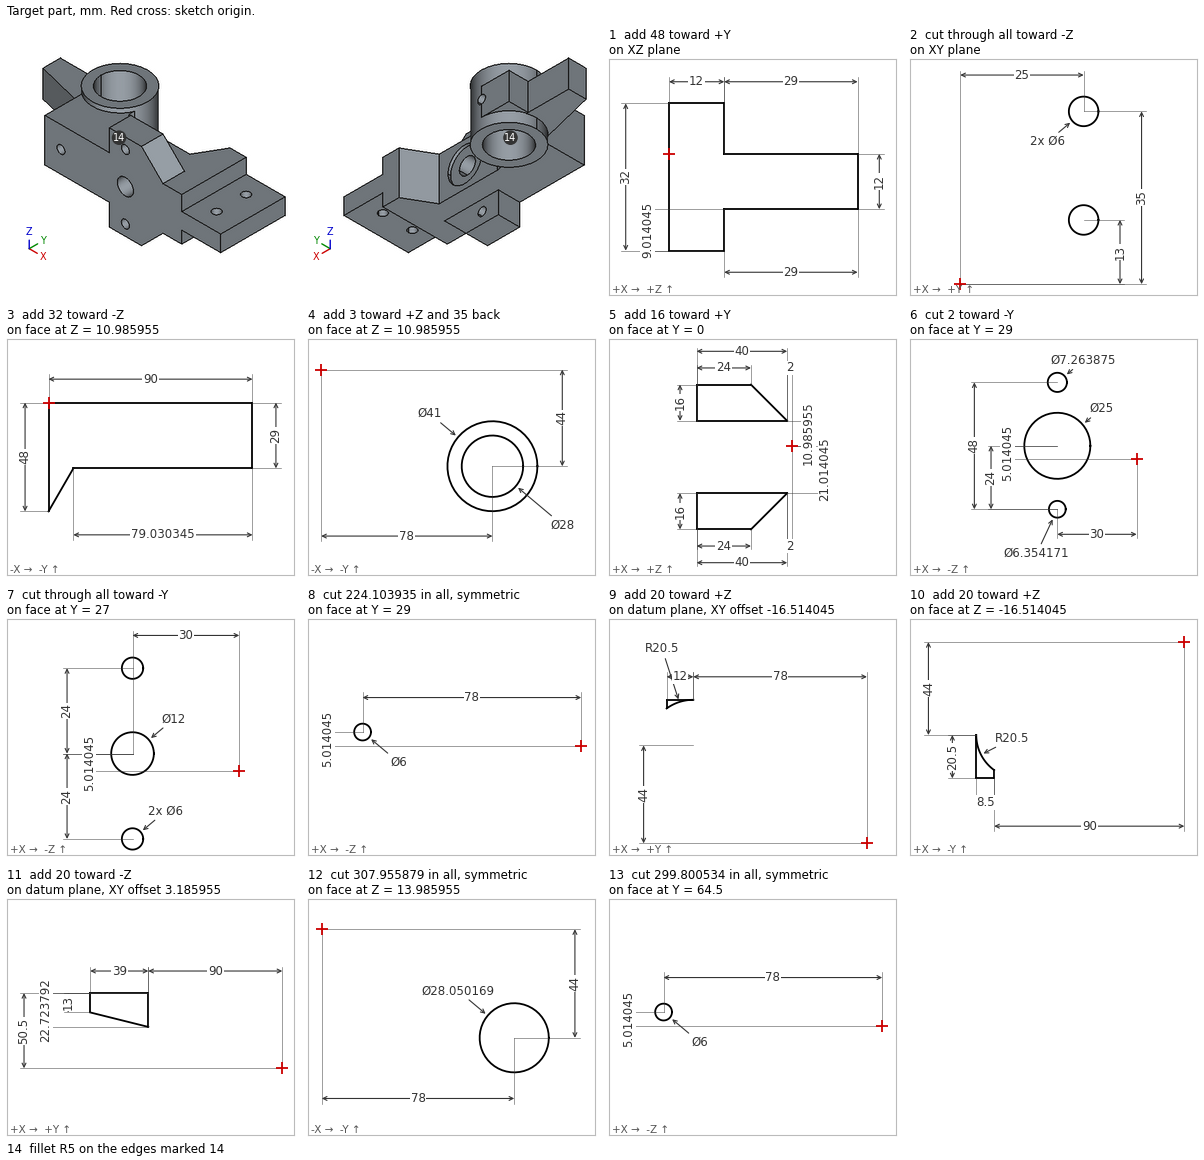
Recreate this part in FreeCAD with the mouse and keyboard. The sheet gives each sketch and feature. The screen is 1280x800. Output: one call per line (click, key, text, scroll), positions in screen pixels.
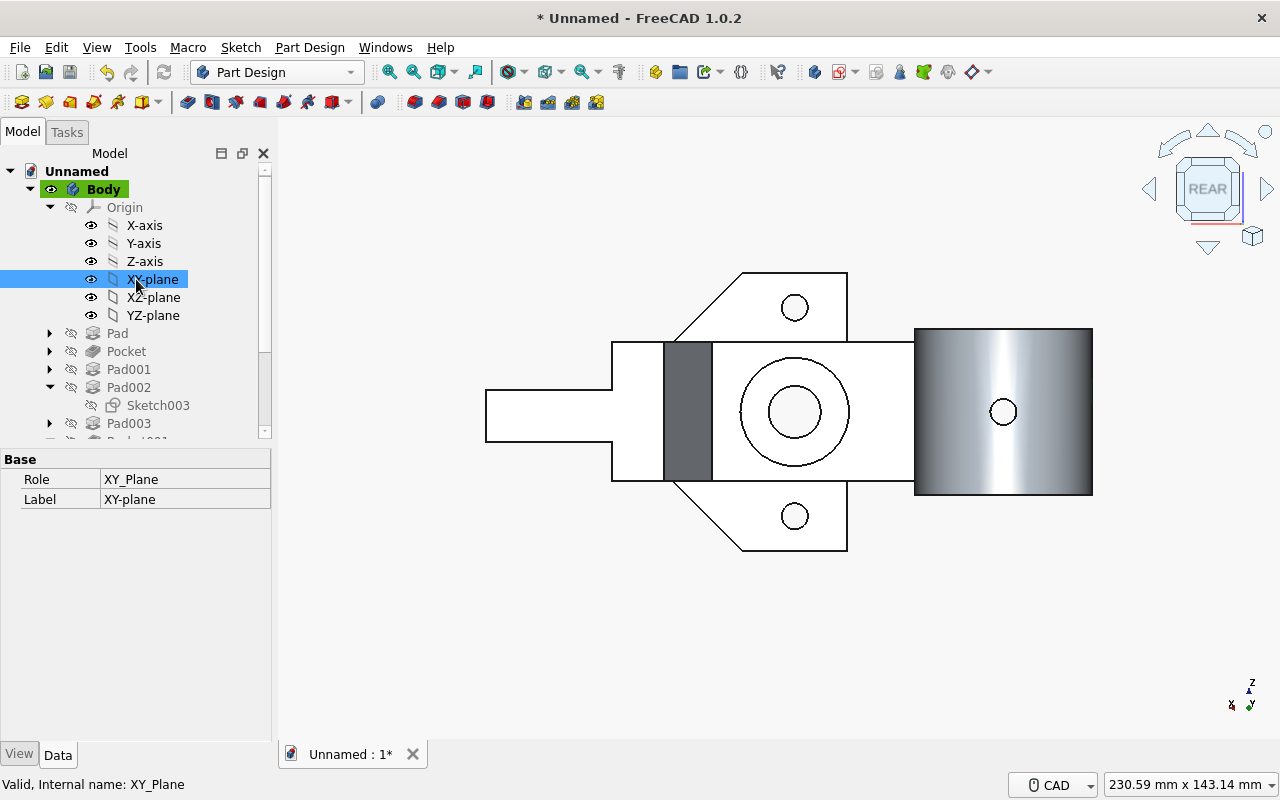
click(972, 72)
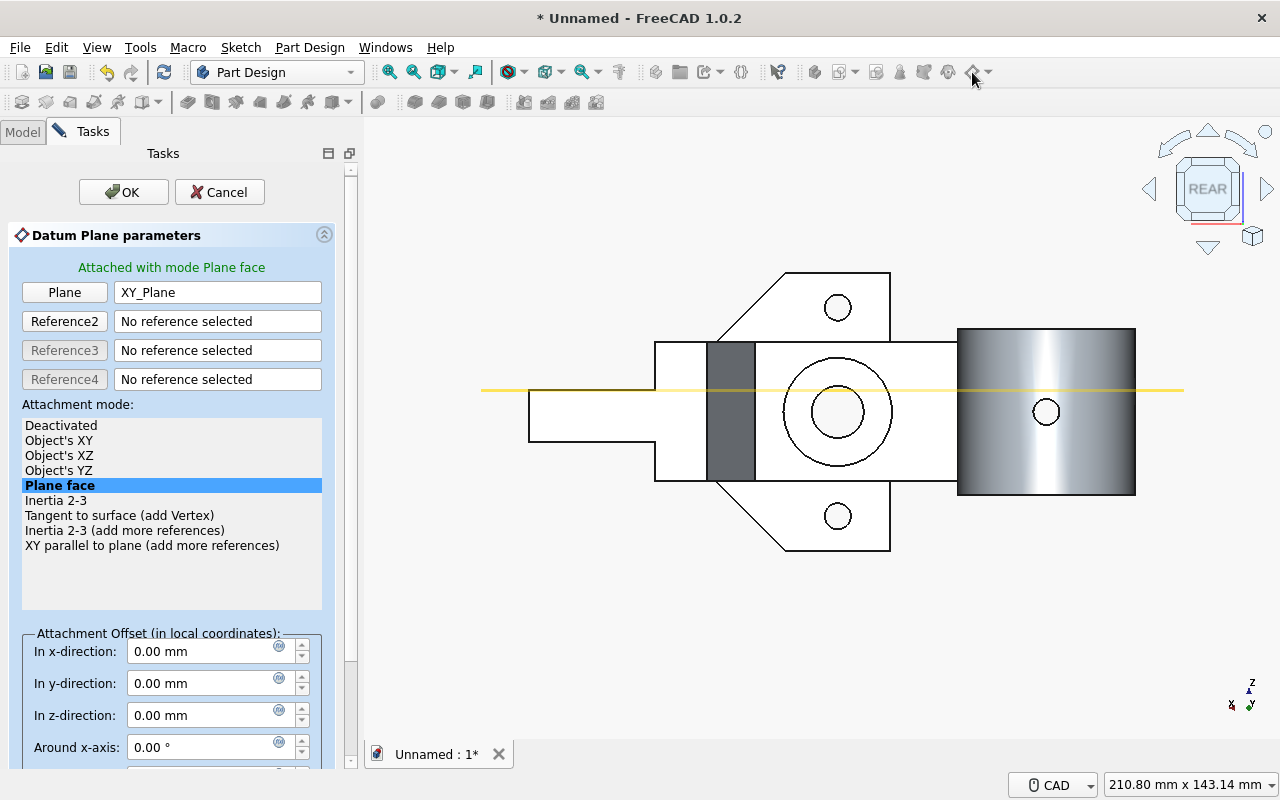
triple_click(210, 715)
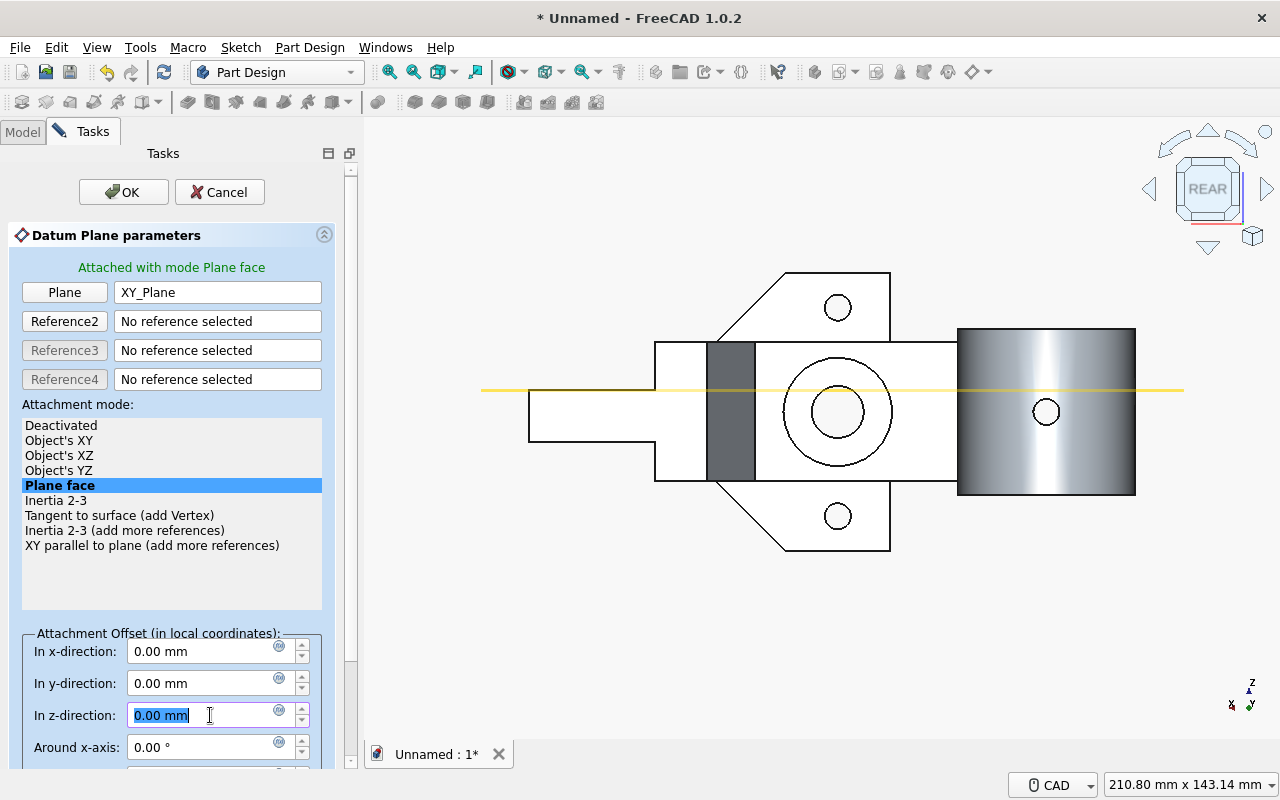
text(-16.514045)
key(Tab)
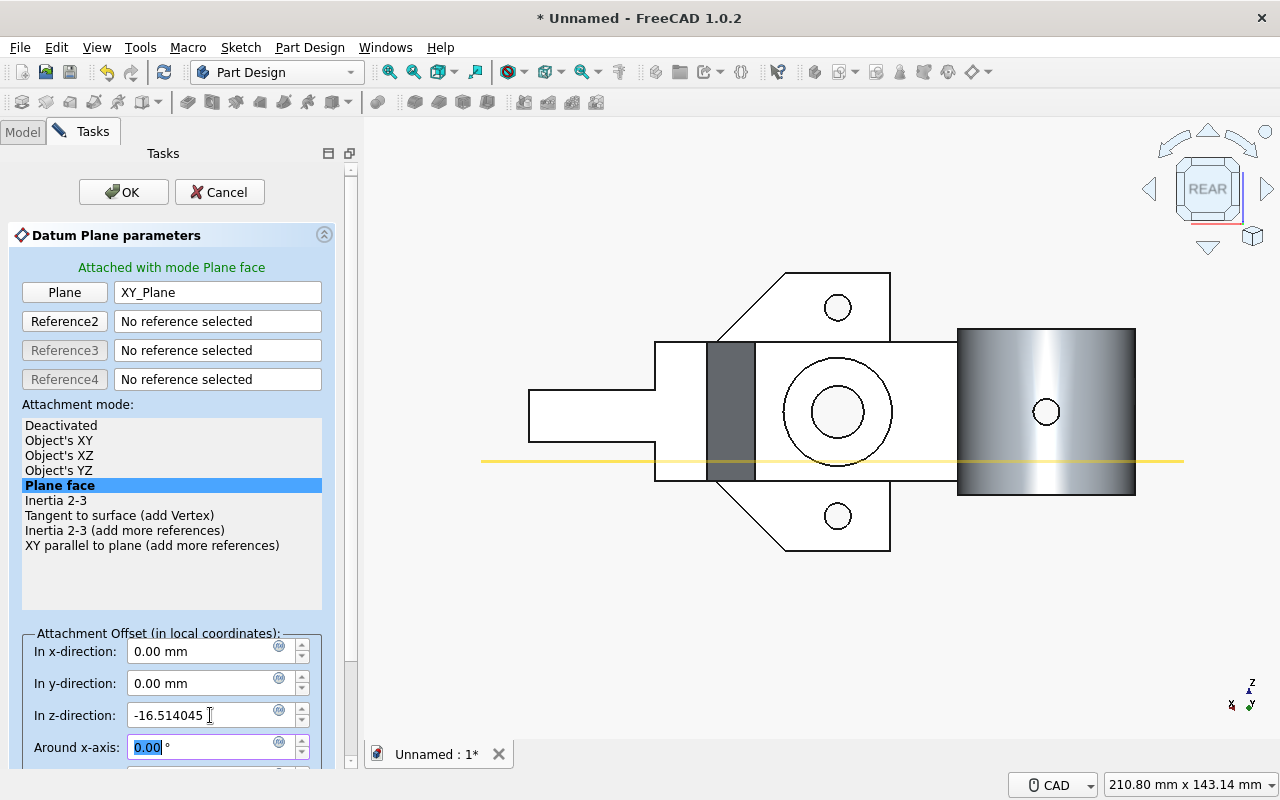
click(124, 192)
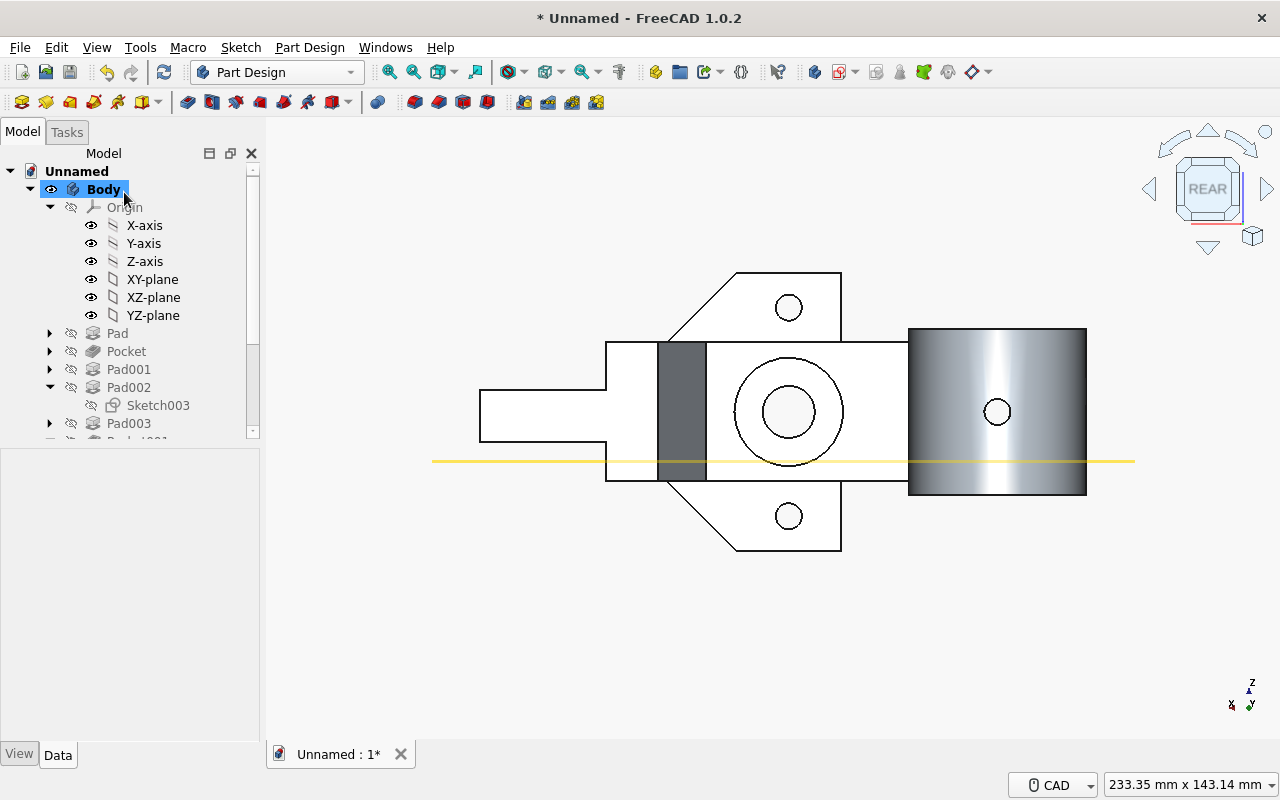
scroll(100, 293, down, 3)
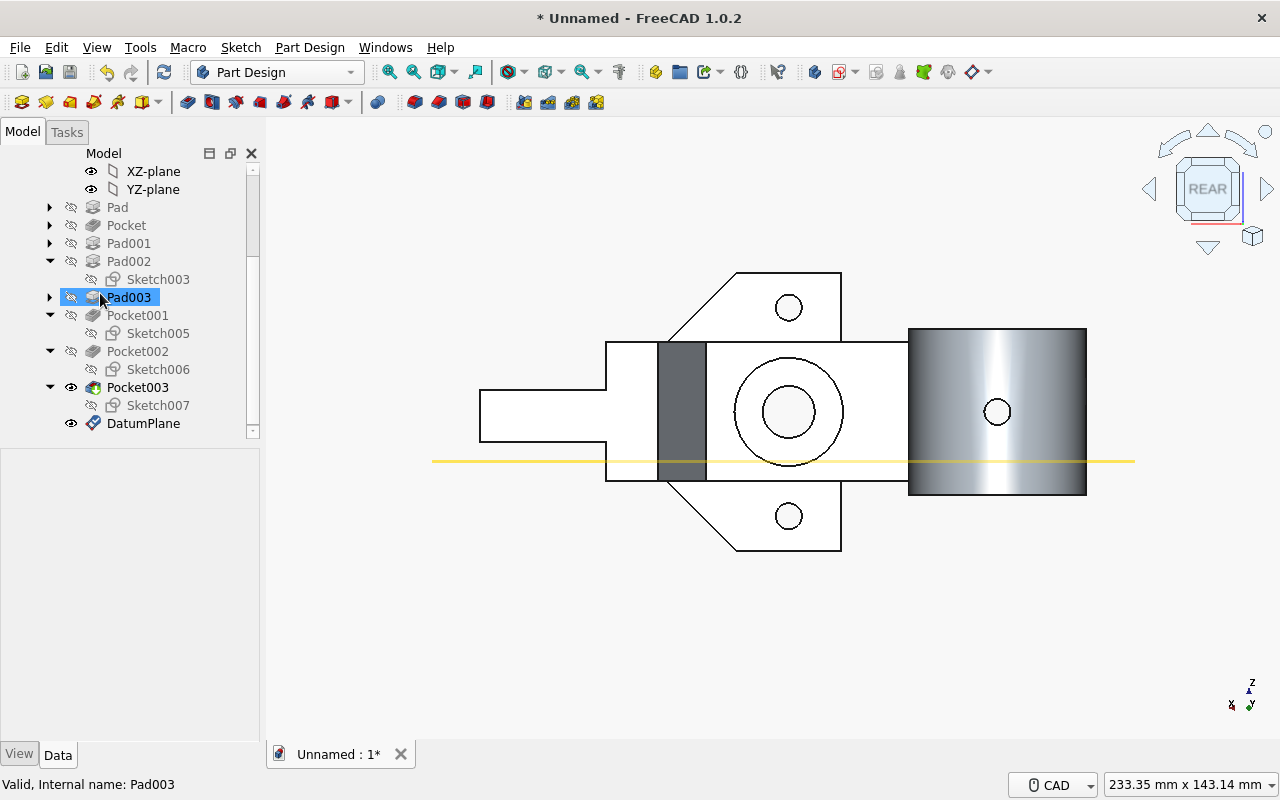
click(116, 423)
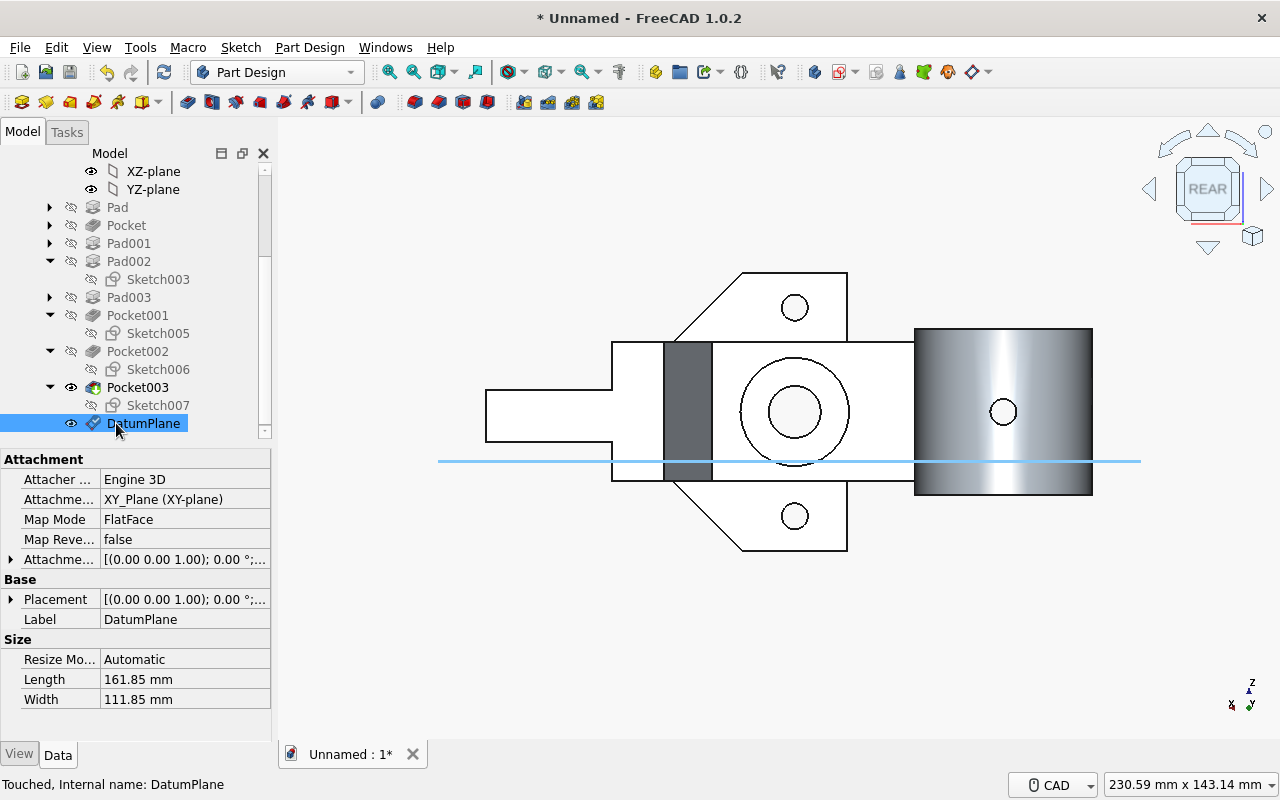
click(840, 72)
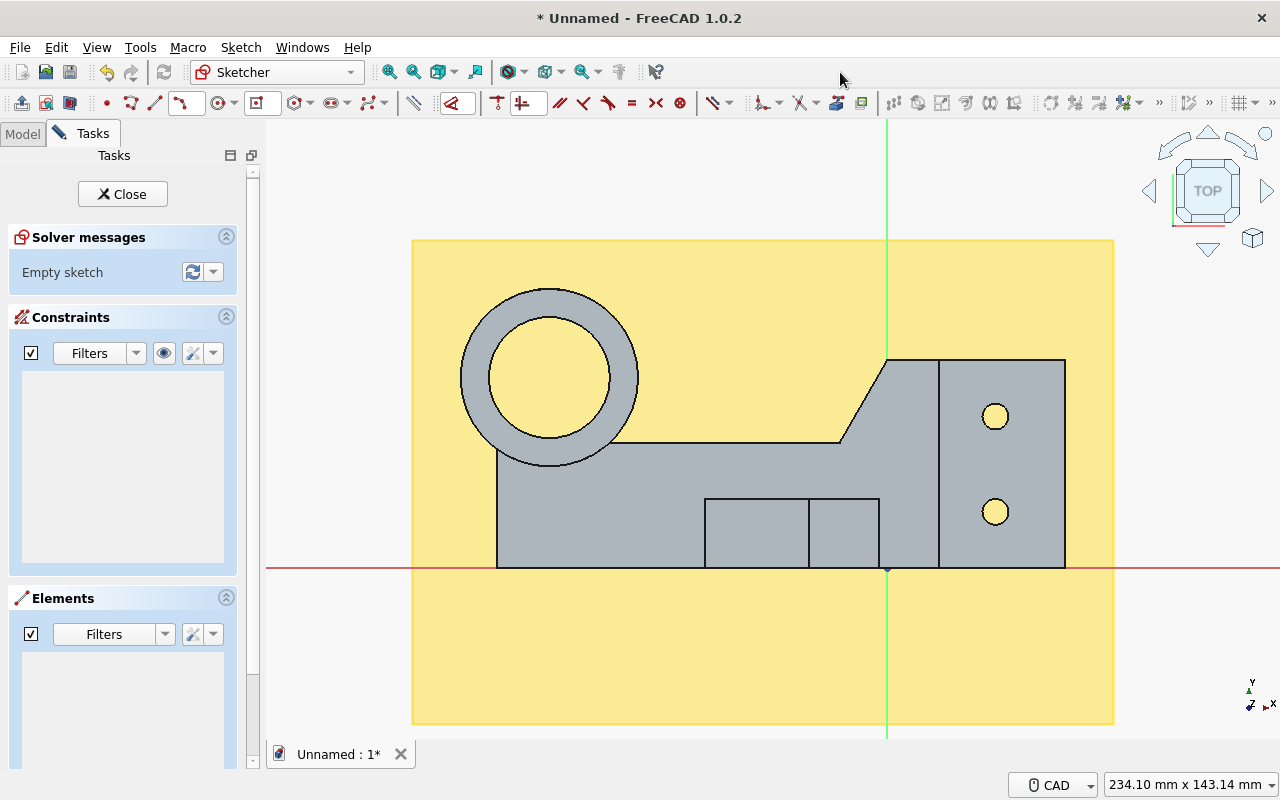
click(70, 104)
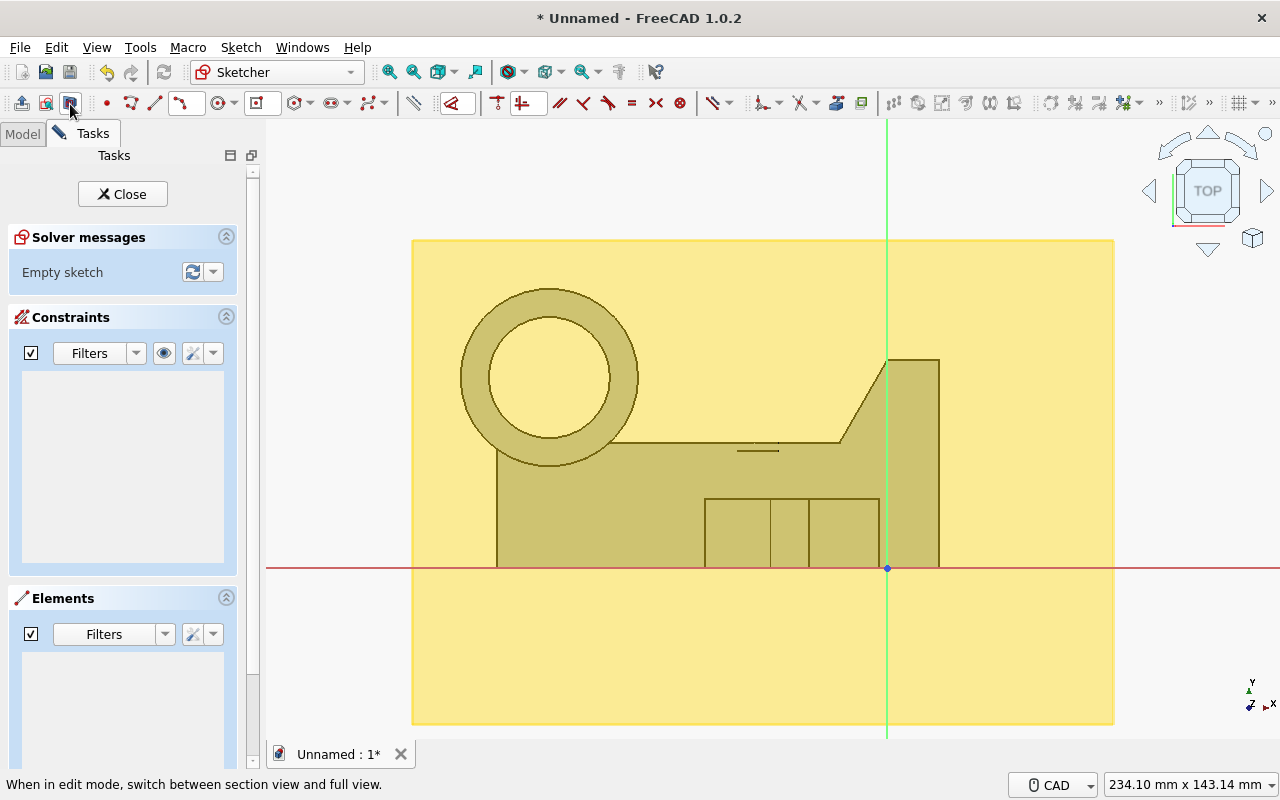
scroll(505, 284, up, 12)